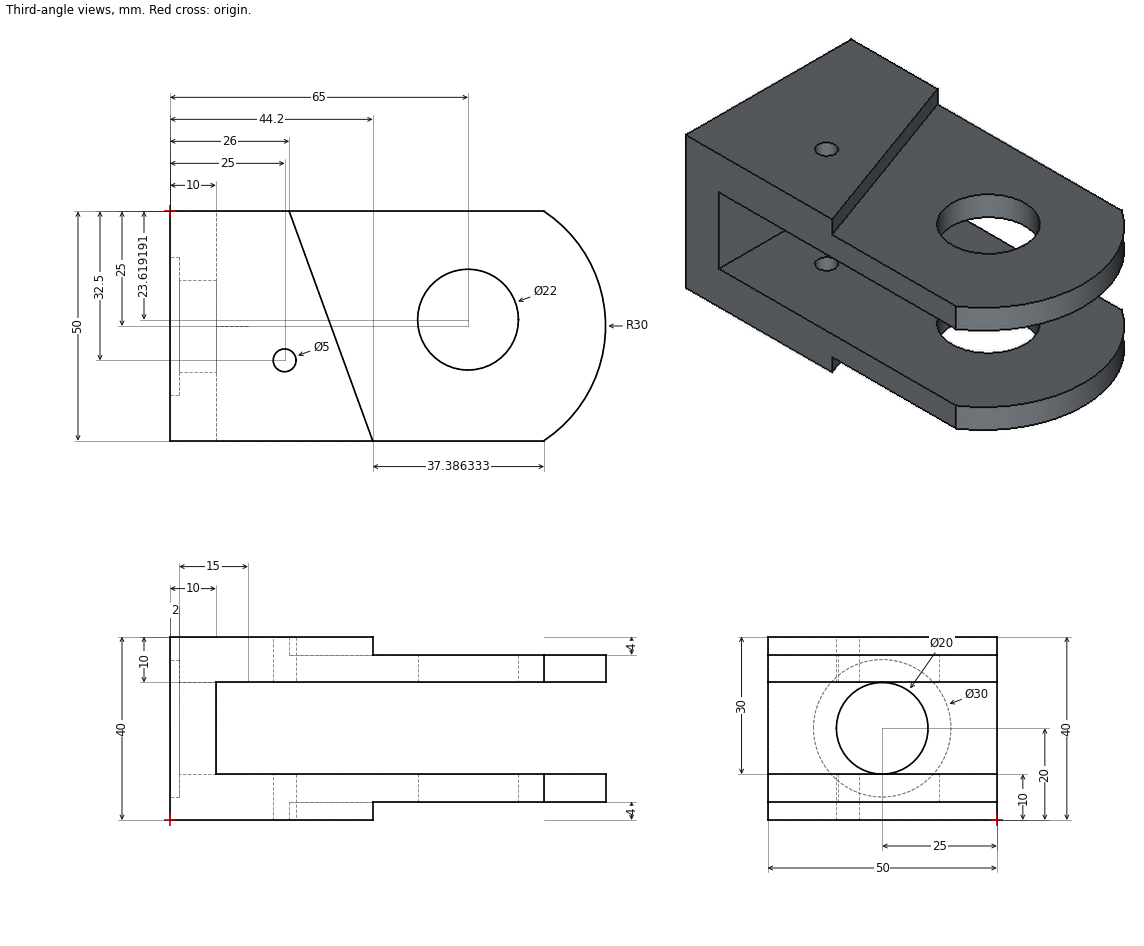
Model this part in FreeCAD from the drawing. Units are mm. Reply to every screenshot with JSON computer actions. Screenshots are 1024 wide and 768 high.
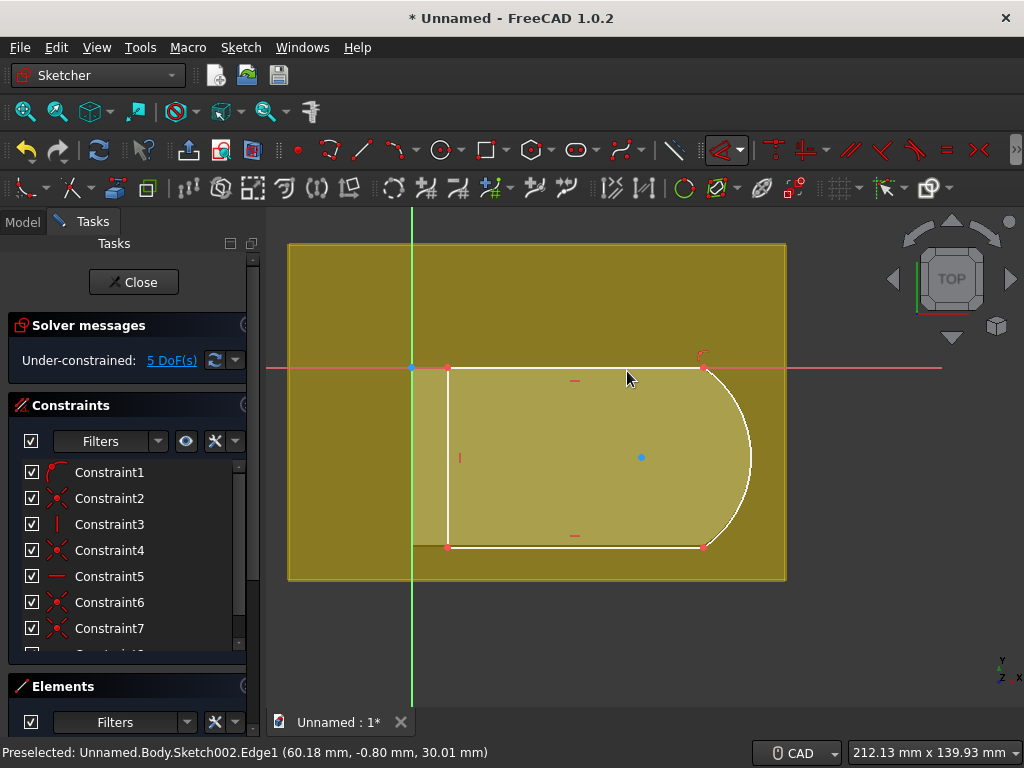
{"action": "left_click", "coordinate": [743, 499]}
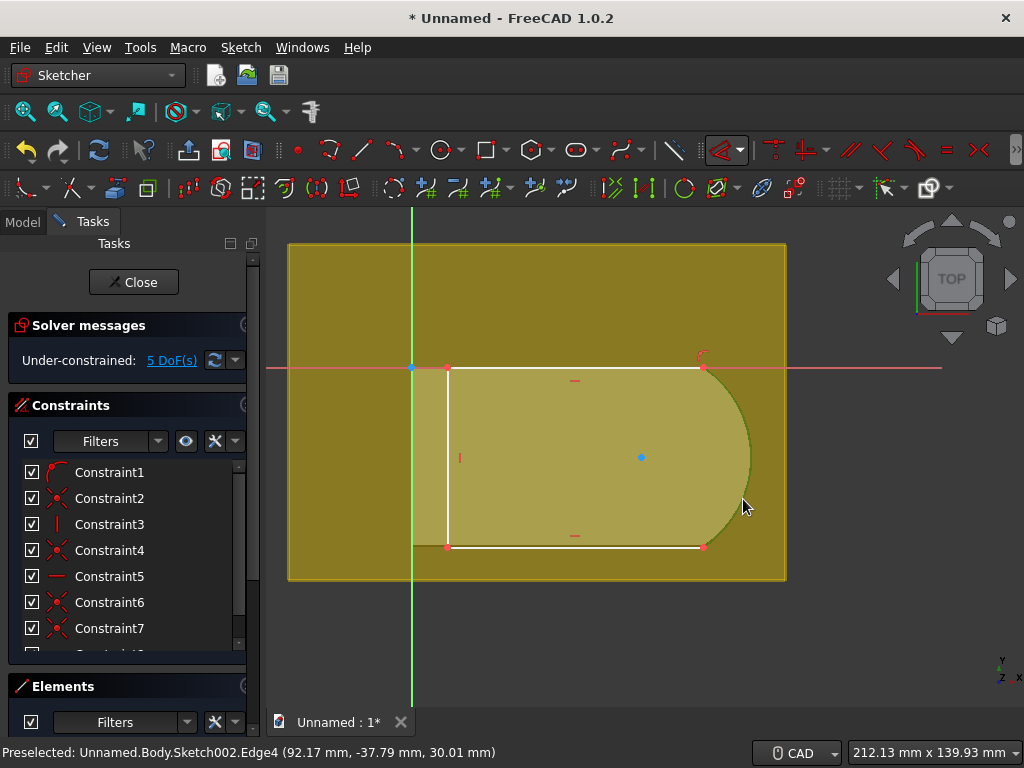
{"action": "key", "text": "k r"}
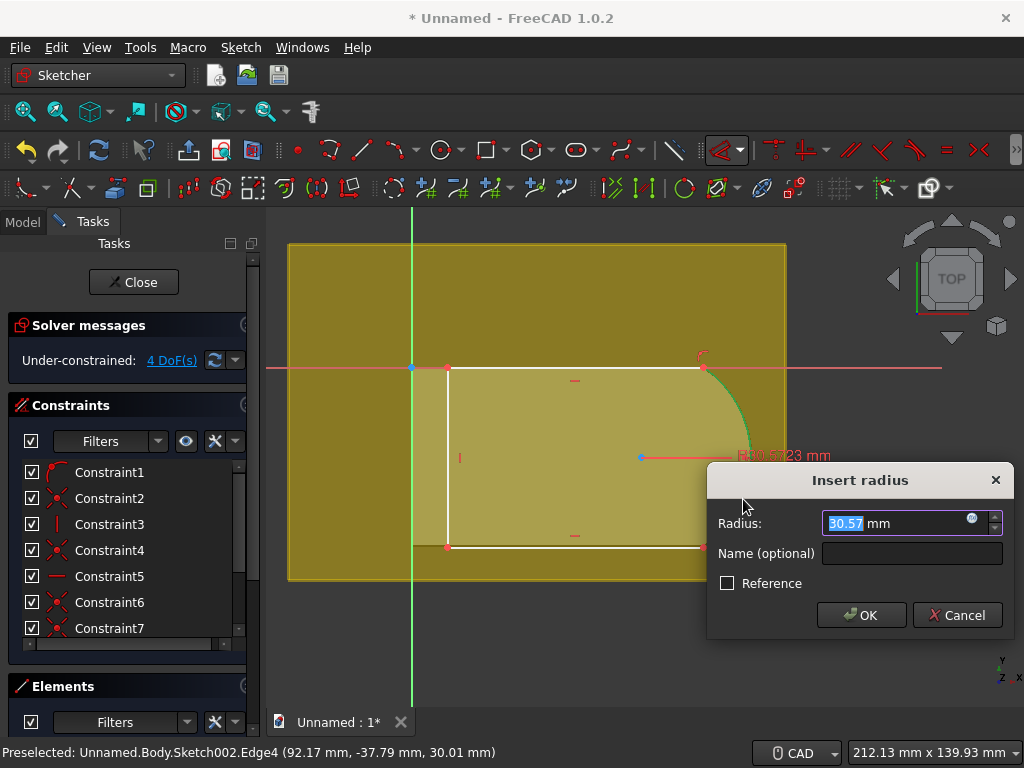
{"action": "type", "text": "30"}
{"action": "key", "text": "Return"}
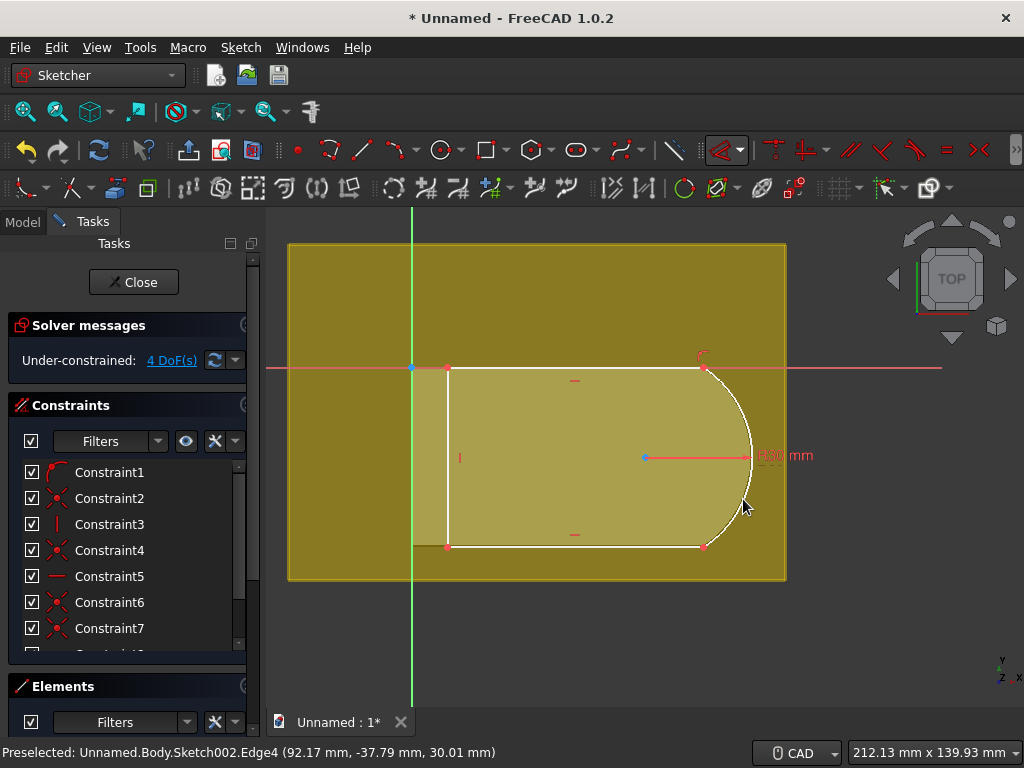
{"action": "left_click", "coordinate": [448, 422]}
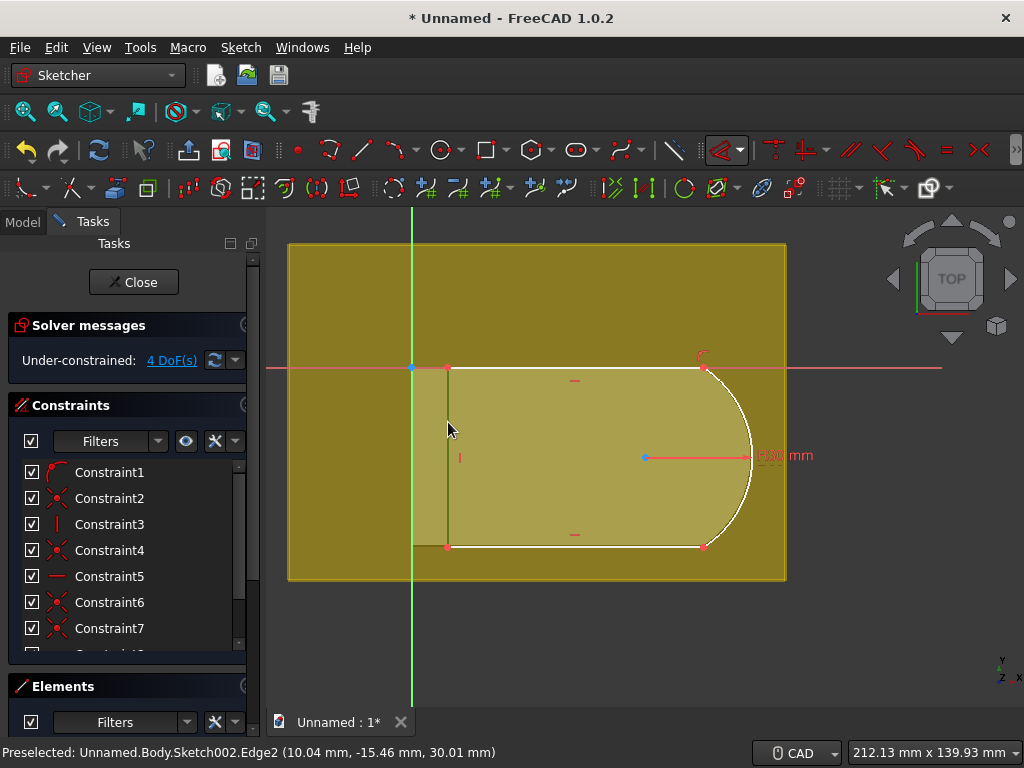
{"action": "key", "text": "i"}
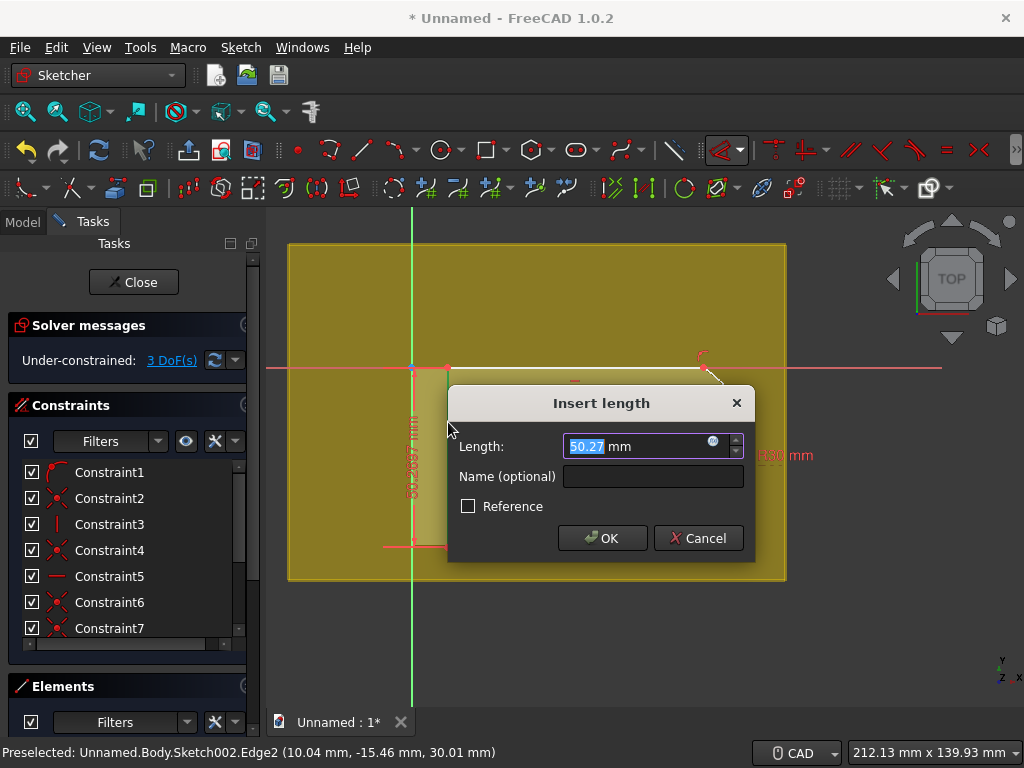
{"action": "type", "text": "50"}
{"action": "key", "text": "Return"}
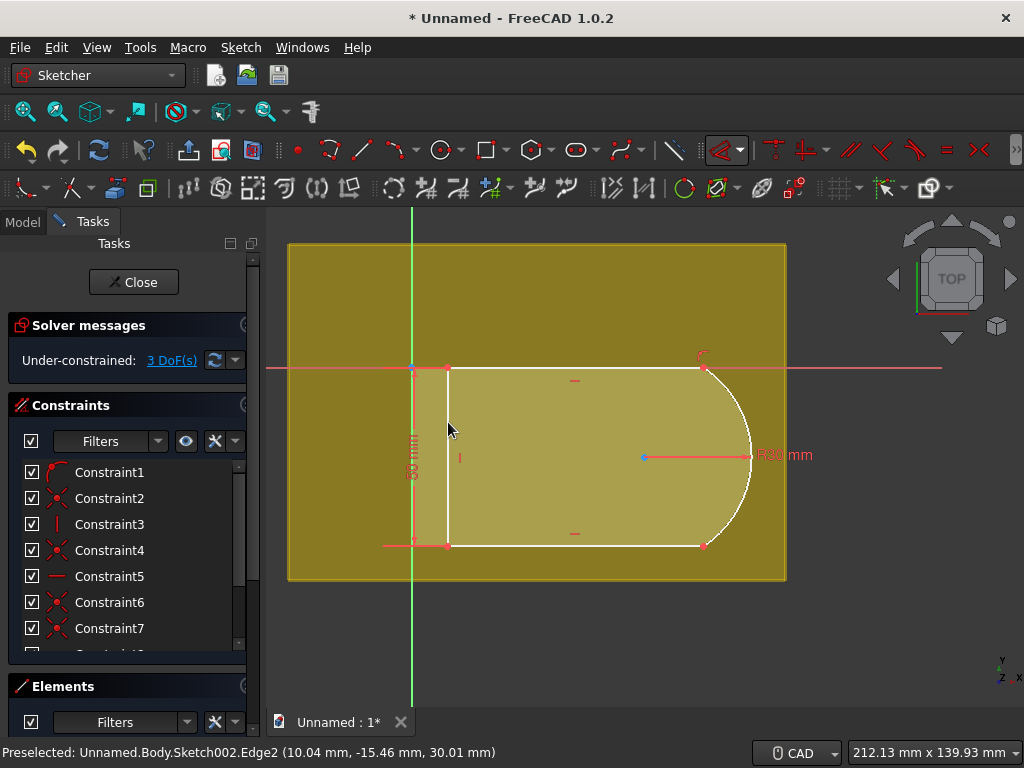
{"action": "left_click", "coordinate": [448, 368]}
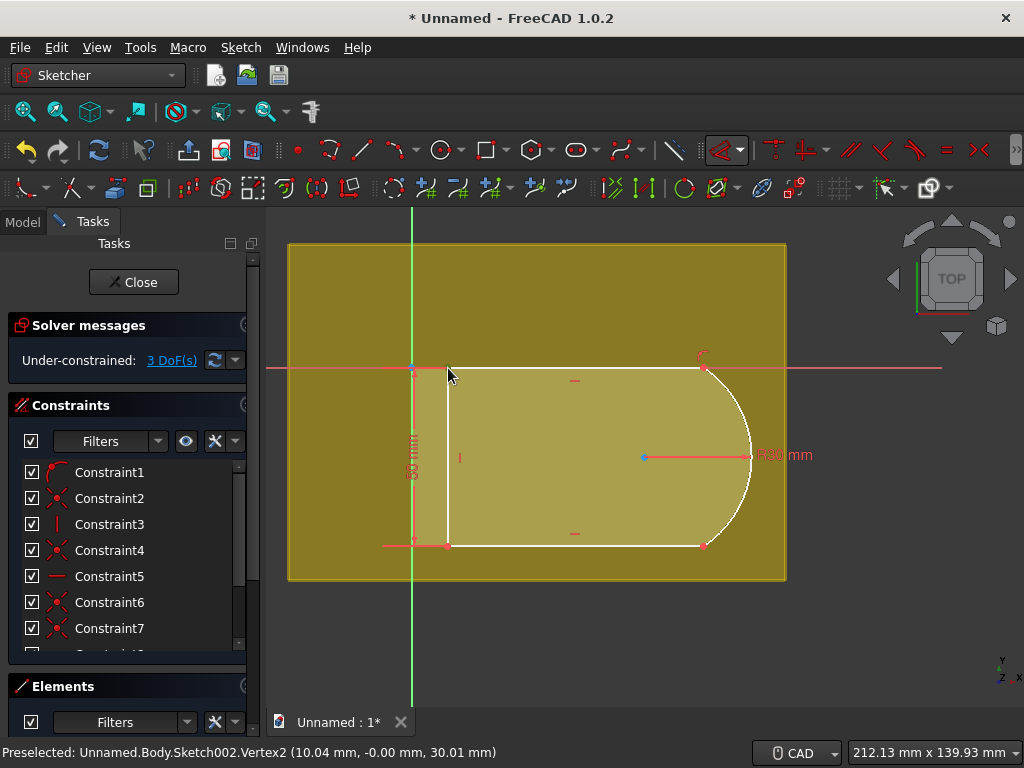
{"action": "key", "text": "l"}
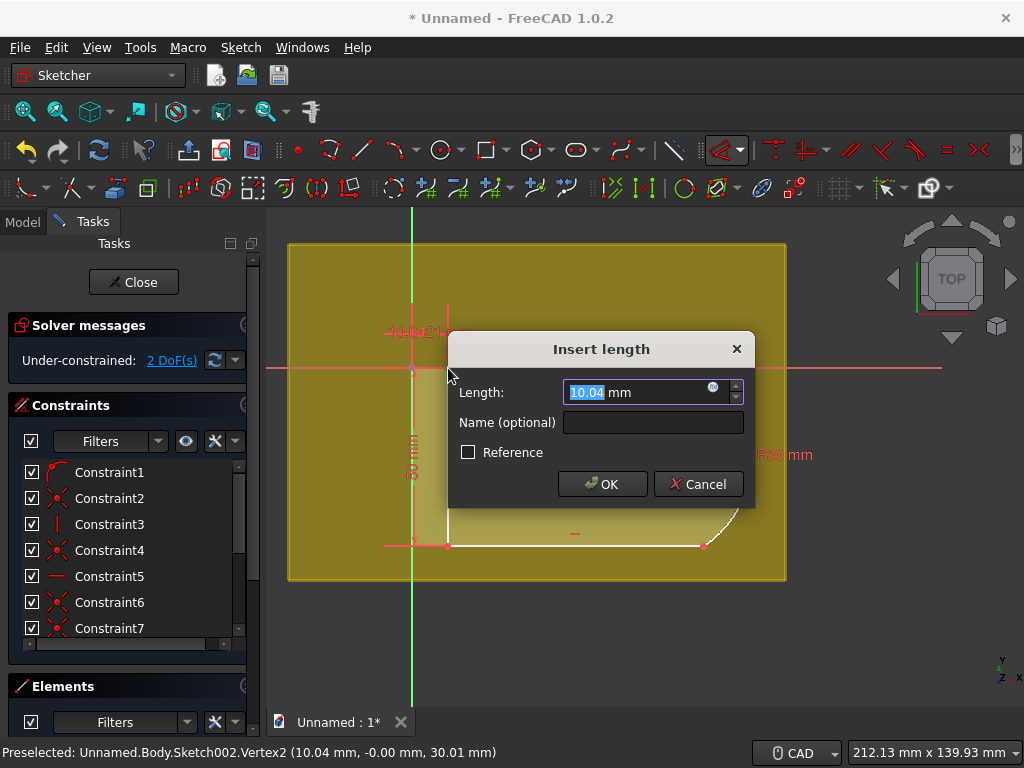
{"action": "type", "text": "10"}
{"action": "key", "text": "Return"}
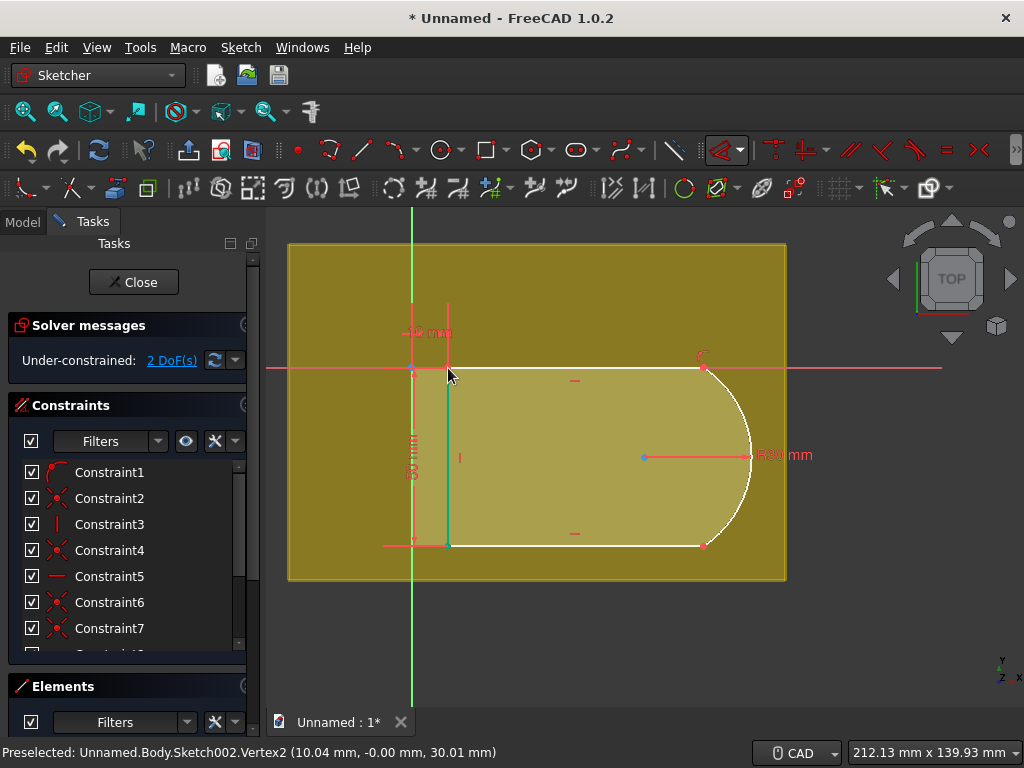
{"action": "left_click", "coordinate": [644, 457]}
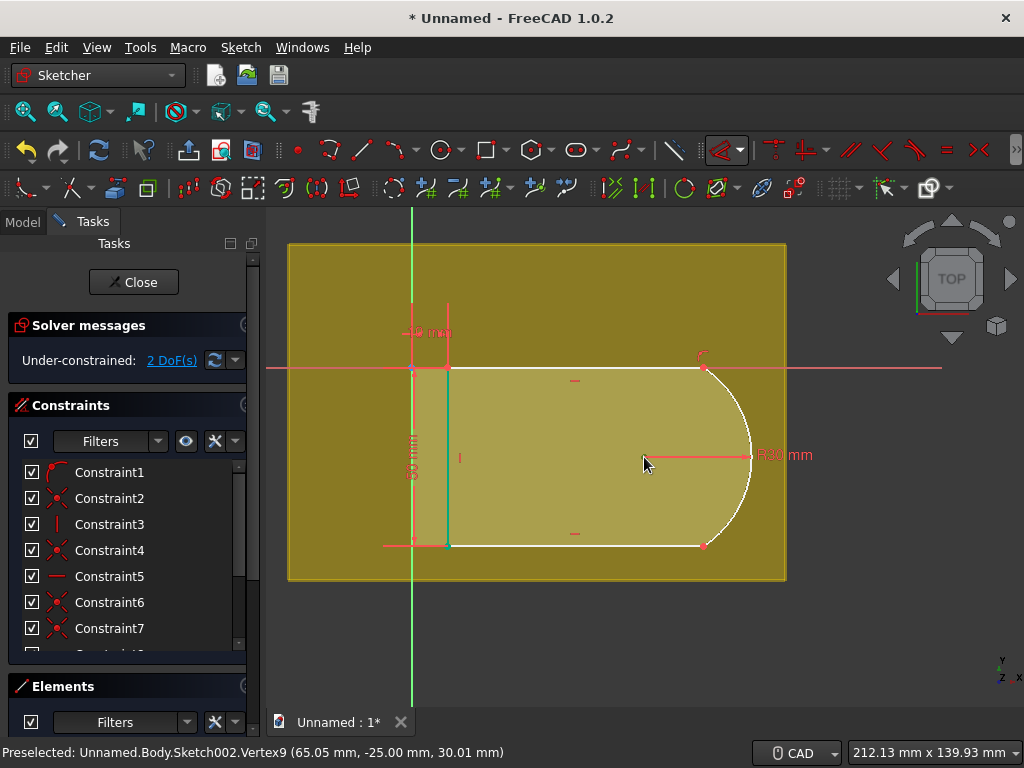
{"action": "left_click", "coordinate": [742, 150]}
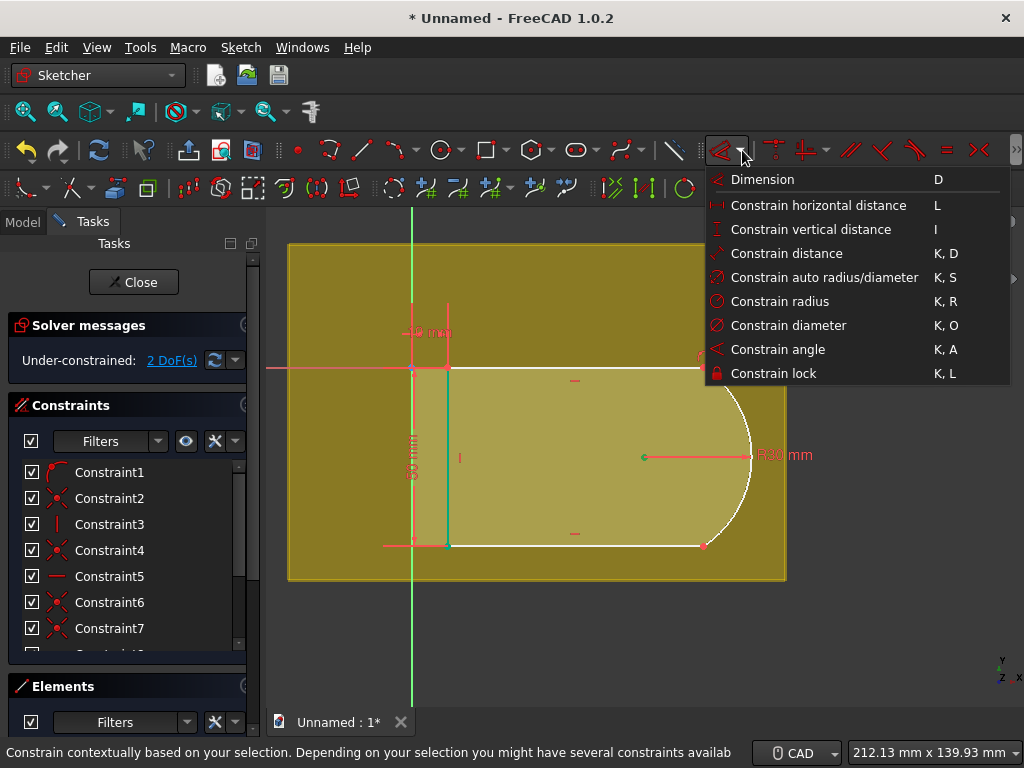
{"action": "left_click", "coordinate": [858, 205]}